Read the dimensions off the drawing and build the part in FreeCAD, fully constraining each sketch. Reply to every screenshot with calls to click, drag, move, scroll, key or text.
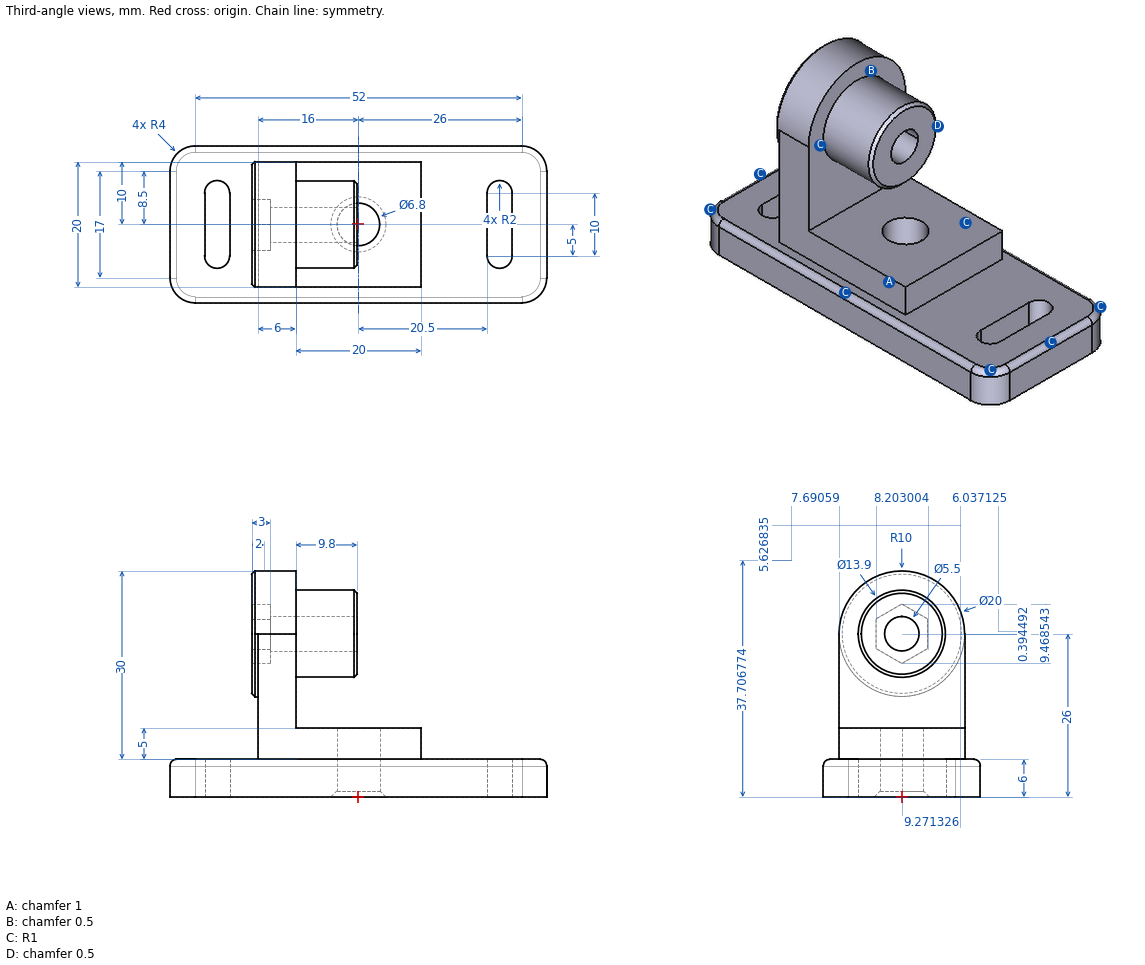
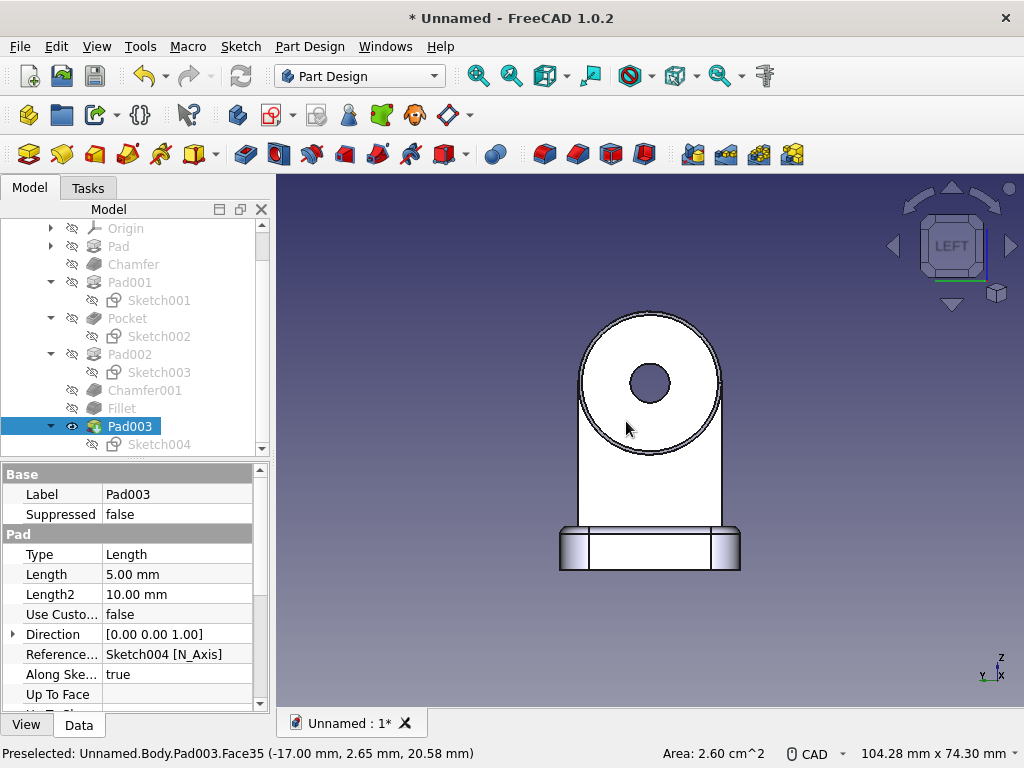
click(270, 116)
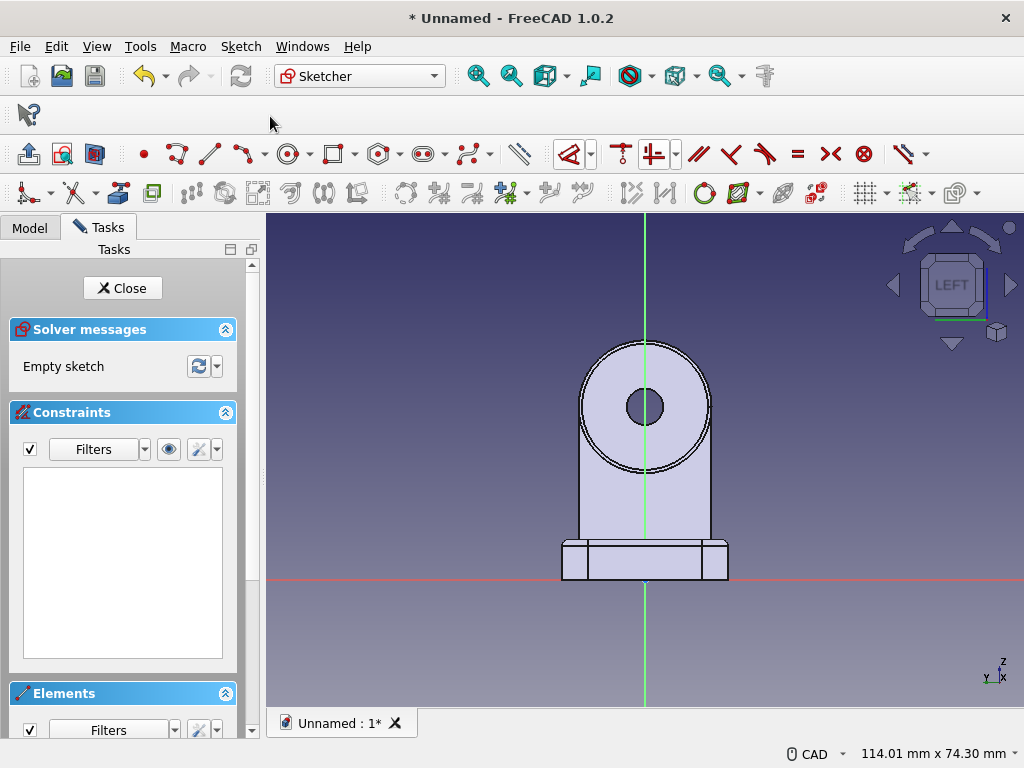
scroll(662, 393, up, 8)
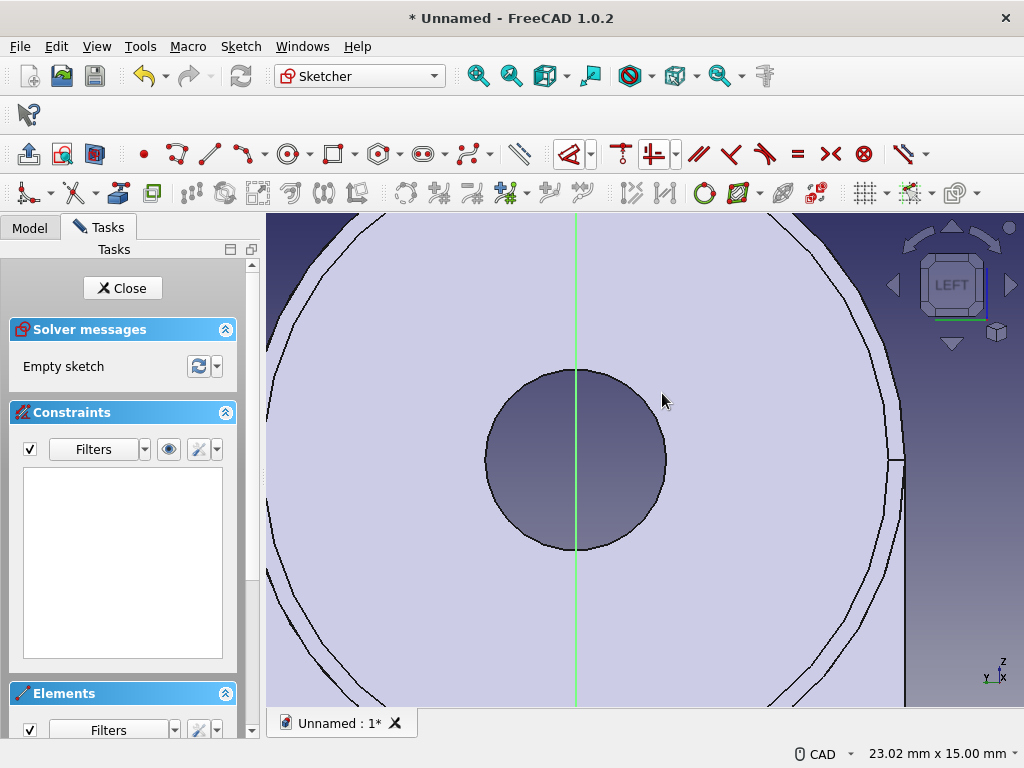
click(378, 154)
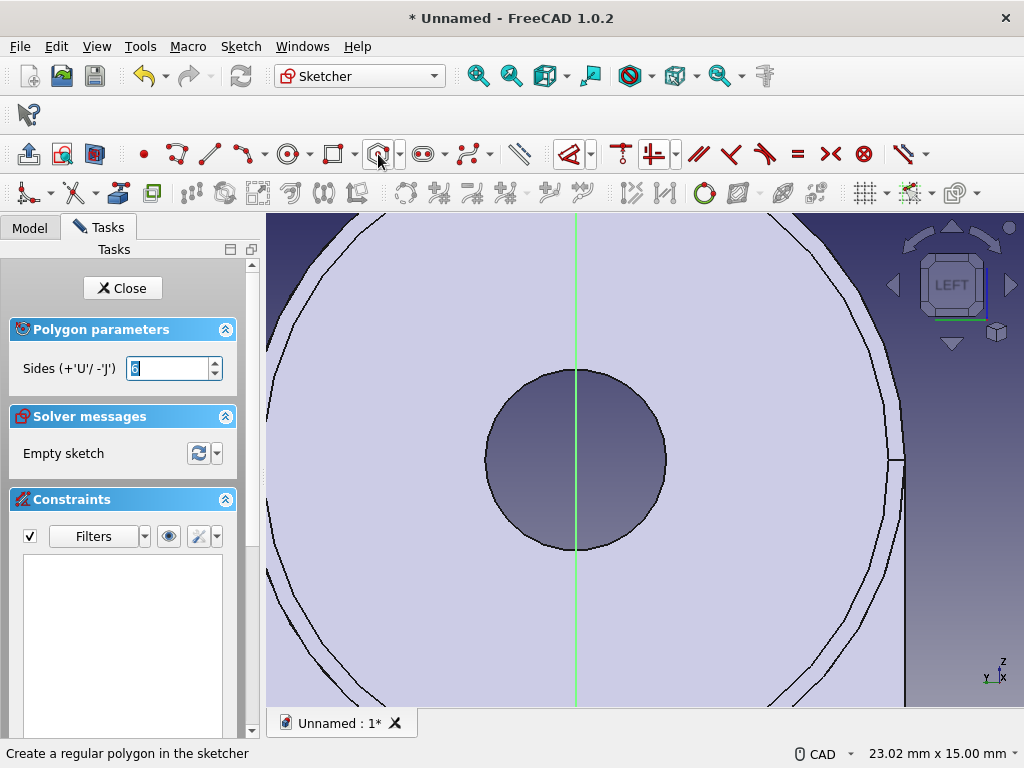
click(576, 460)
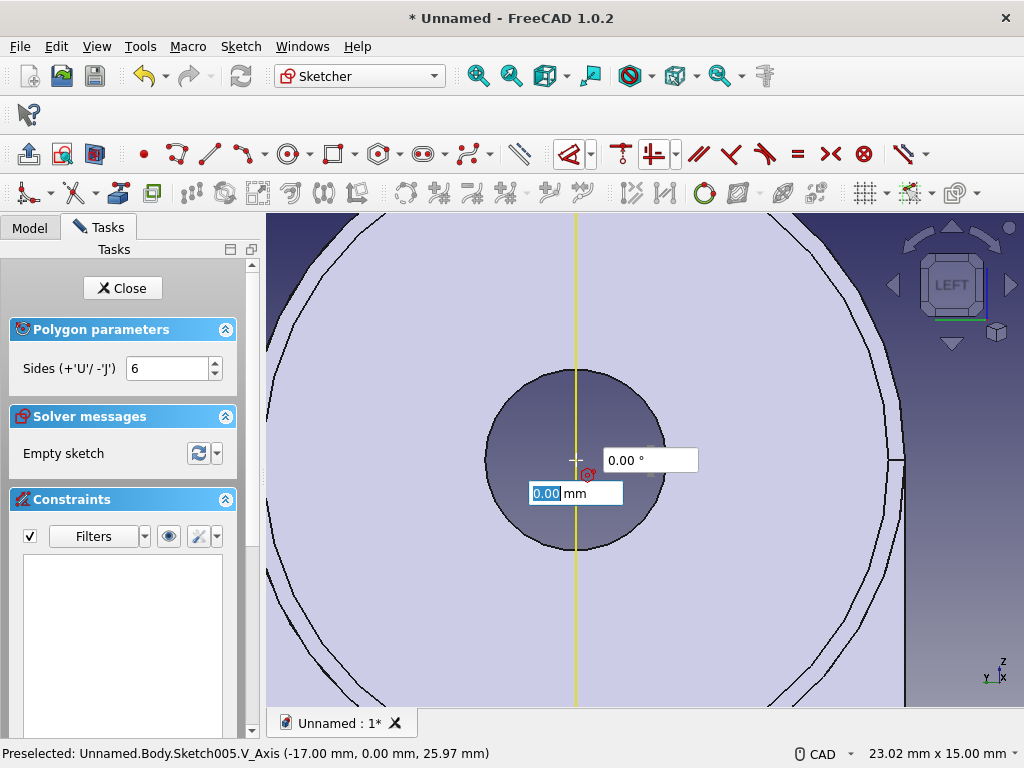
click(441, 538)
right_click(441, 538)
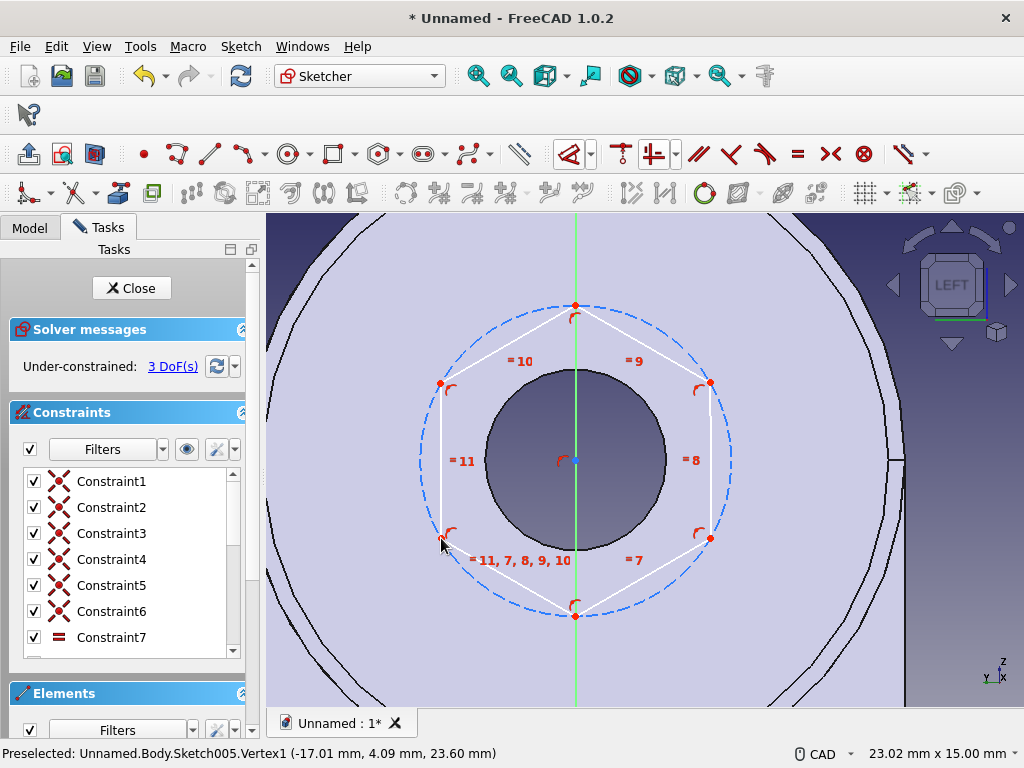
click(576, 461)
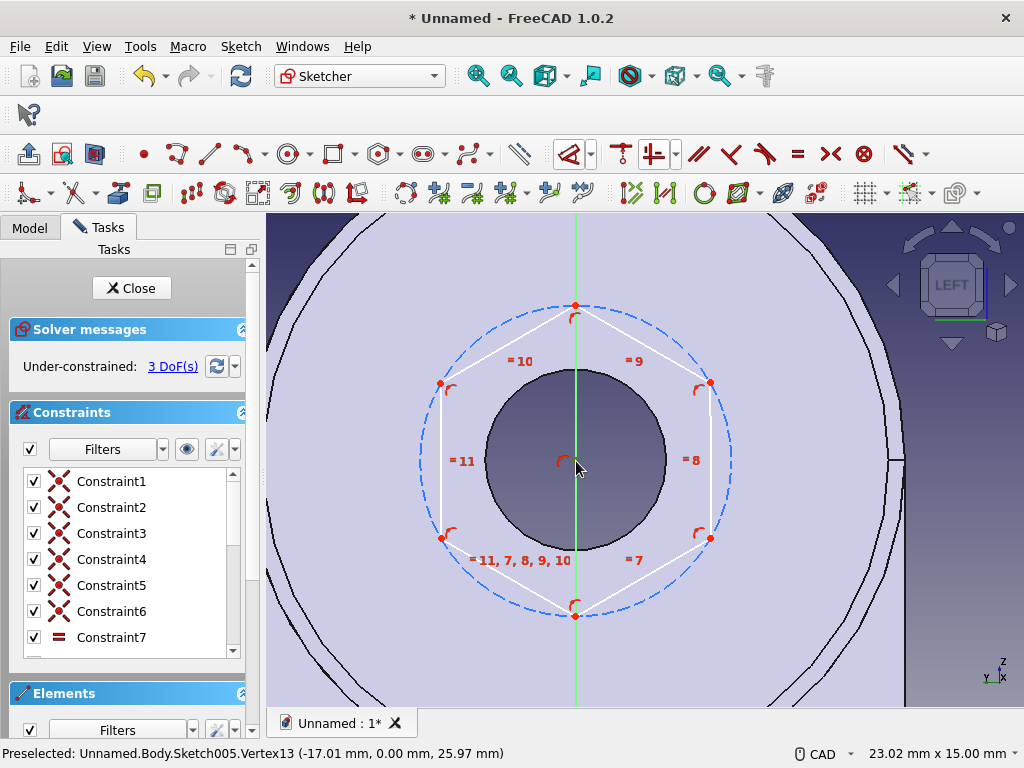
key(i)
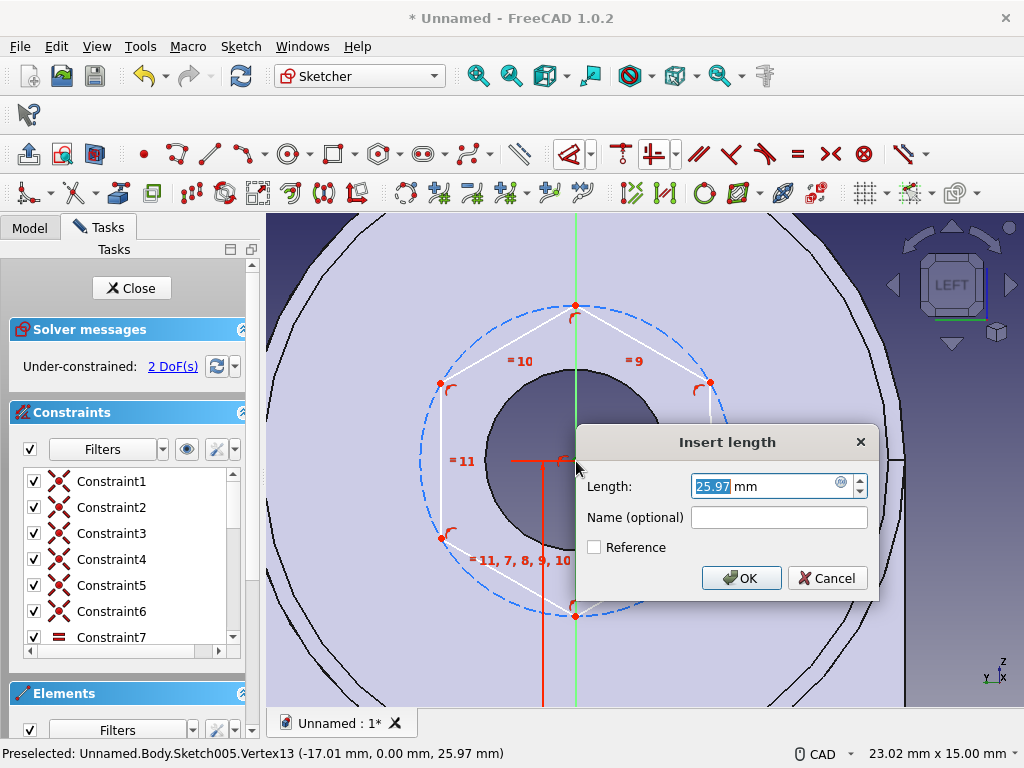
text(26)
key(Return)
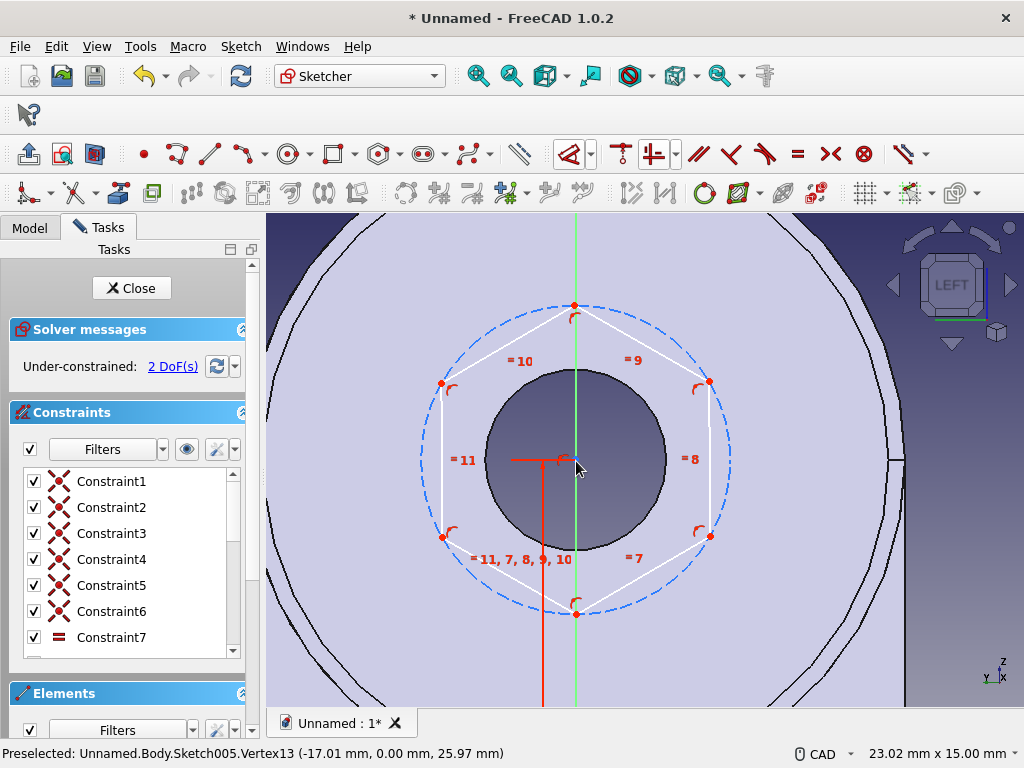
click(442, 538)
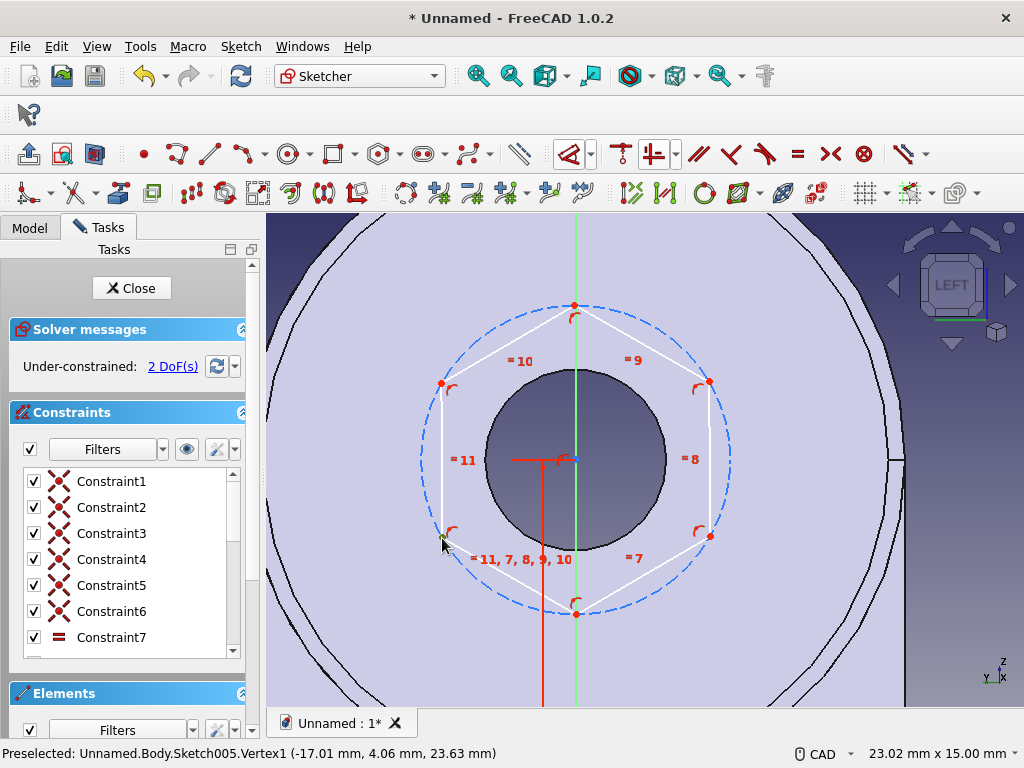
click(709, 382)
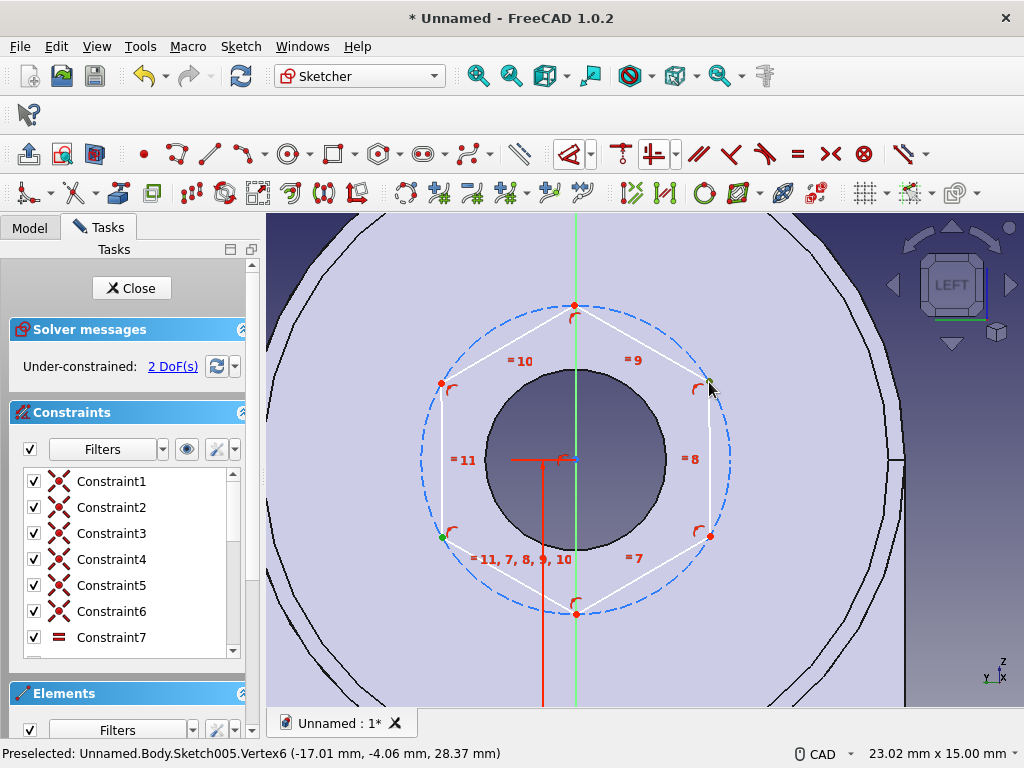
click(590, 154)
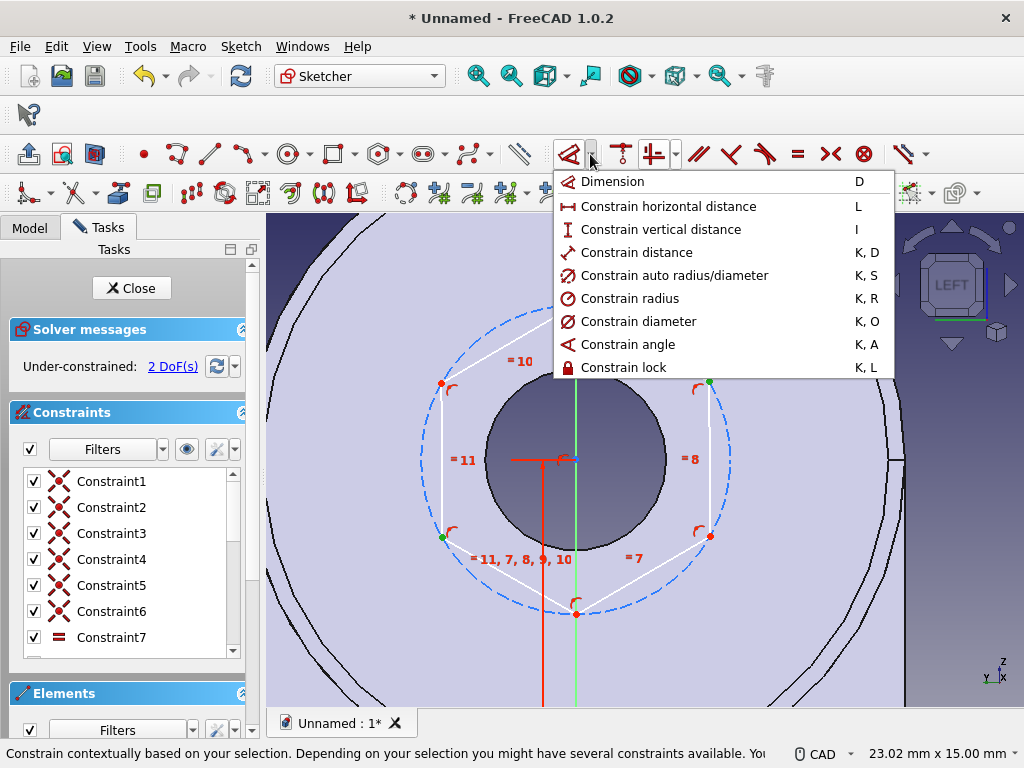
click(724, 206)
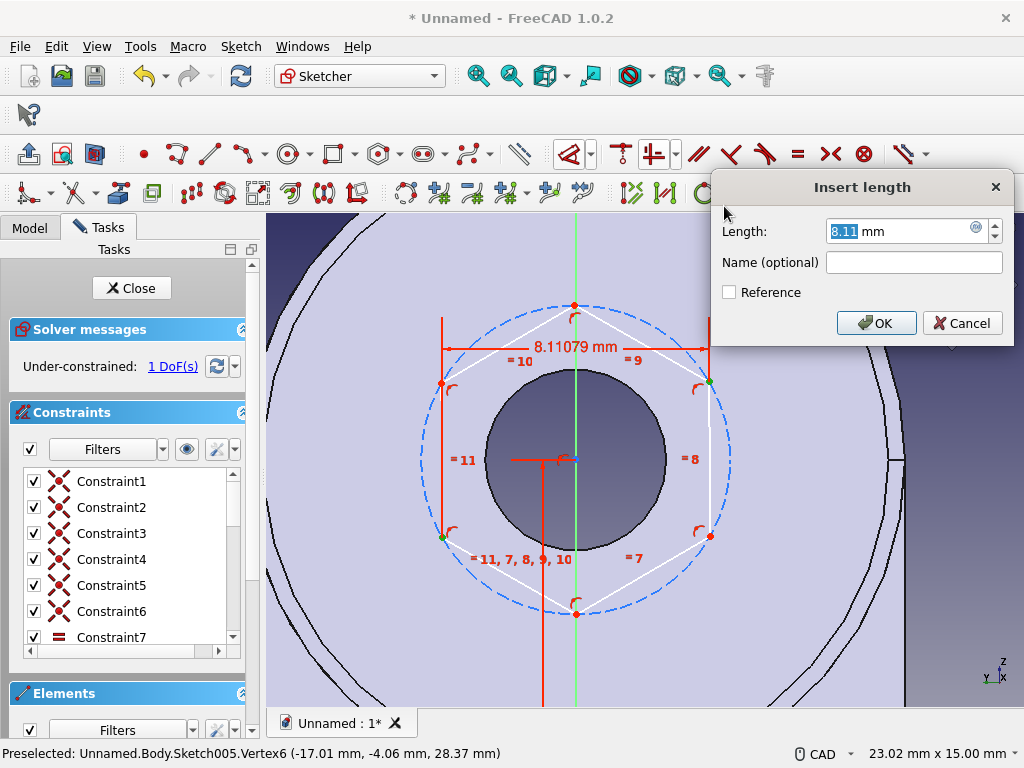
text(8.203004)
key(Return)